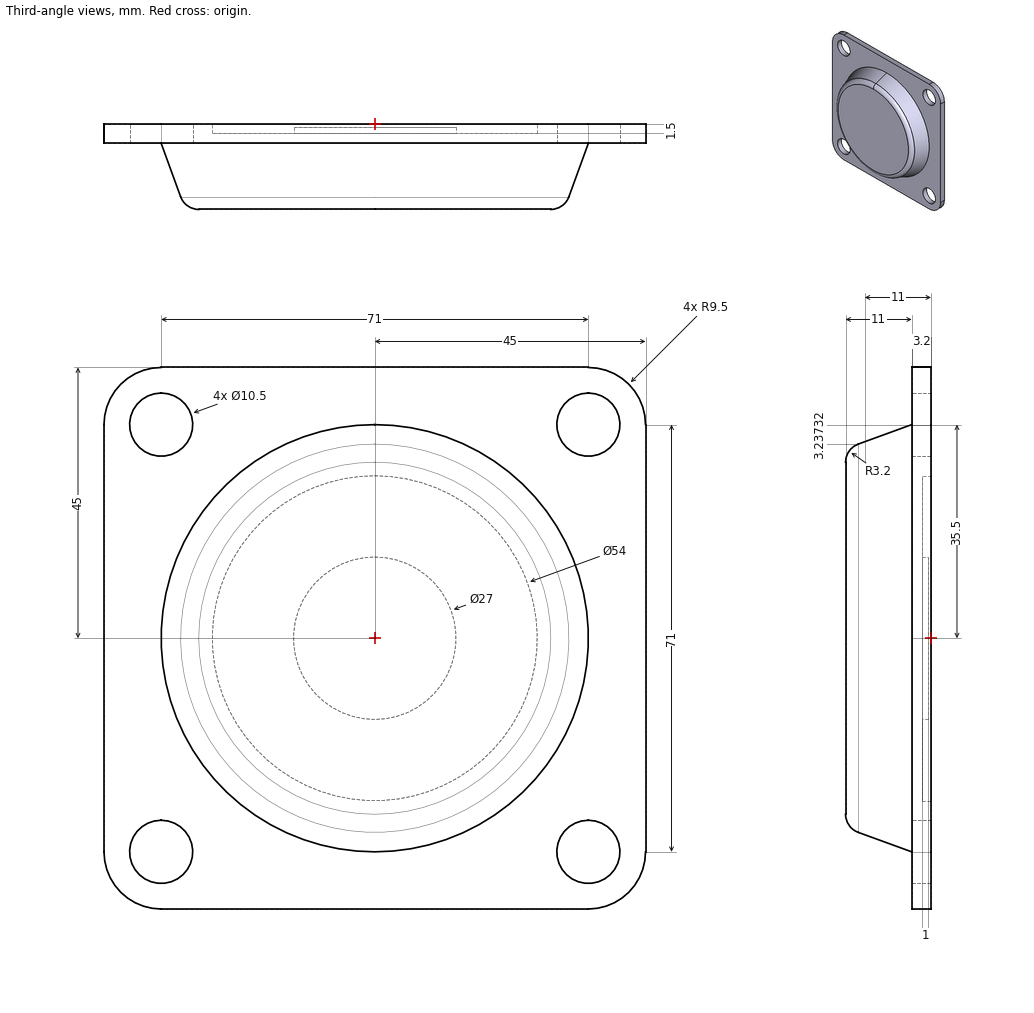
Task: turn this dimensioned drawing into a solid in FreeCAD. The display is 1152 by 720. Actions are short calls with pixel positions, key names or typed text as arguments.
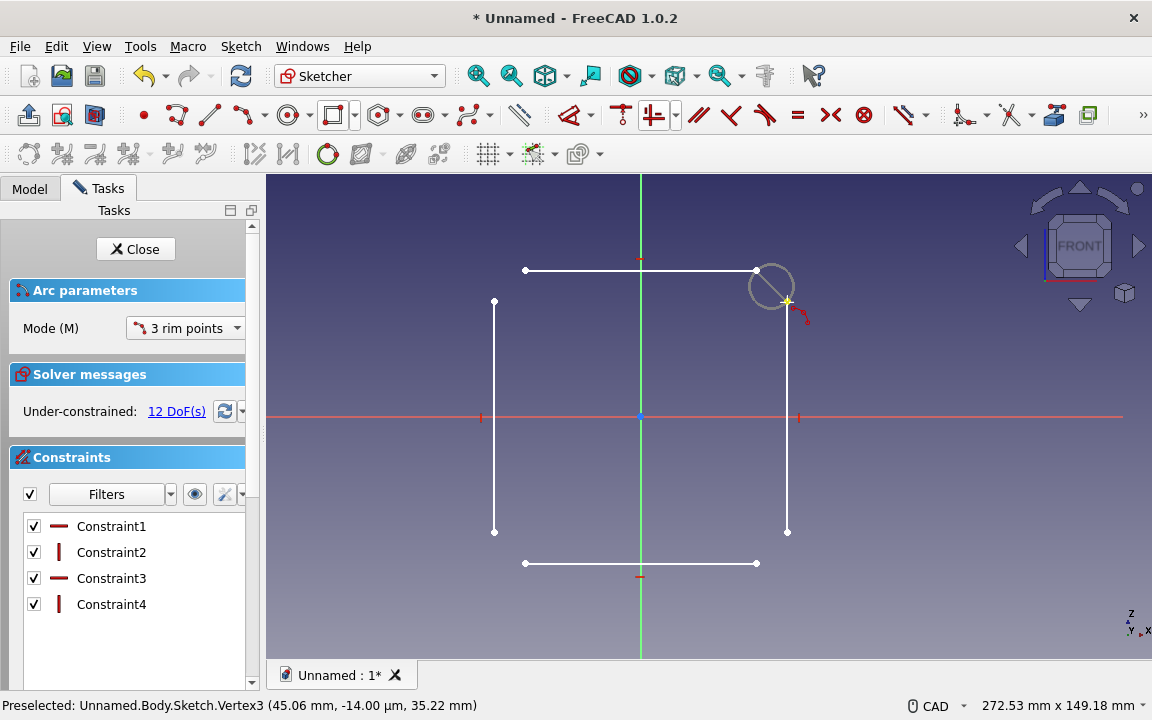
scroll(778, 279, up, 3)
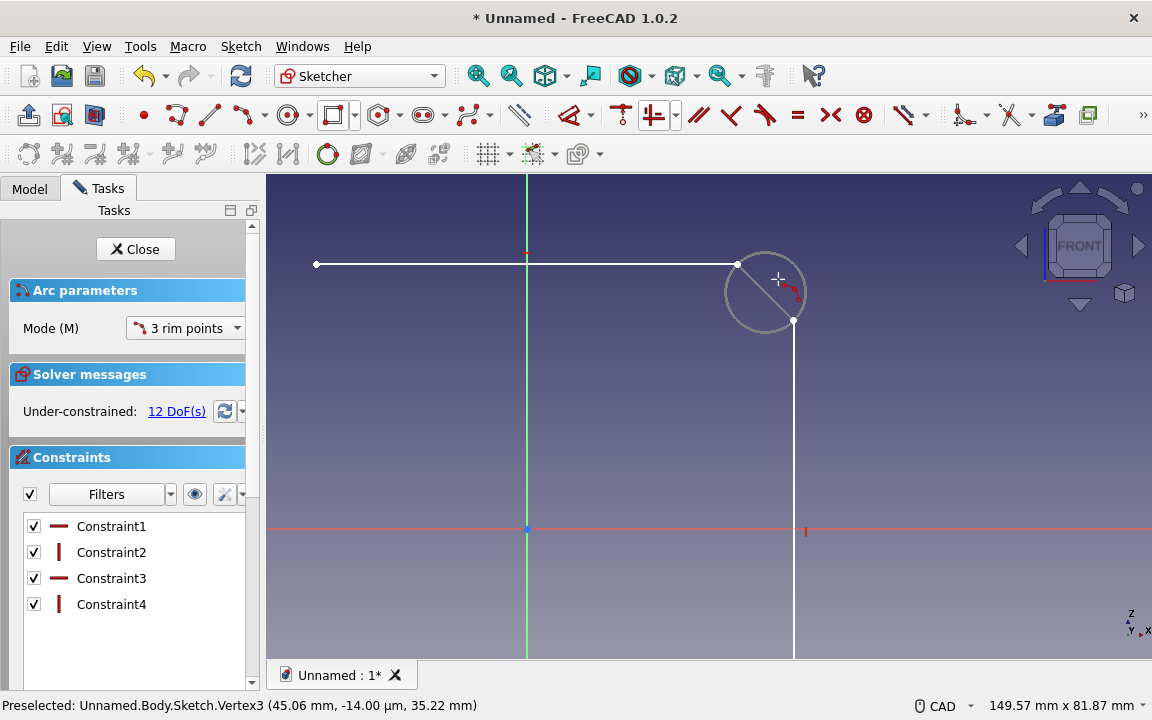
click(777, 279)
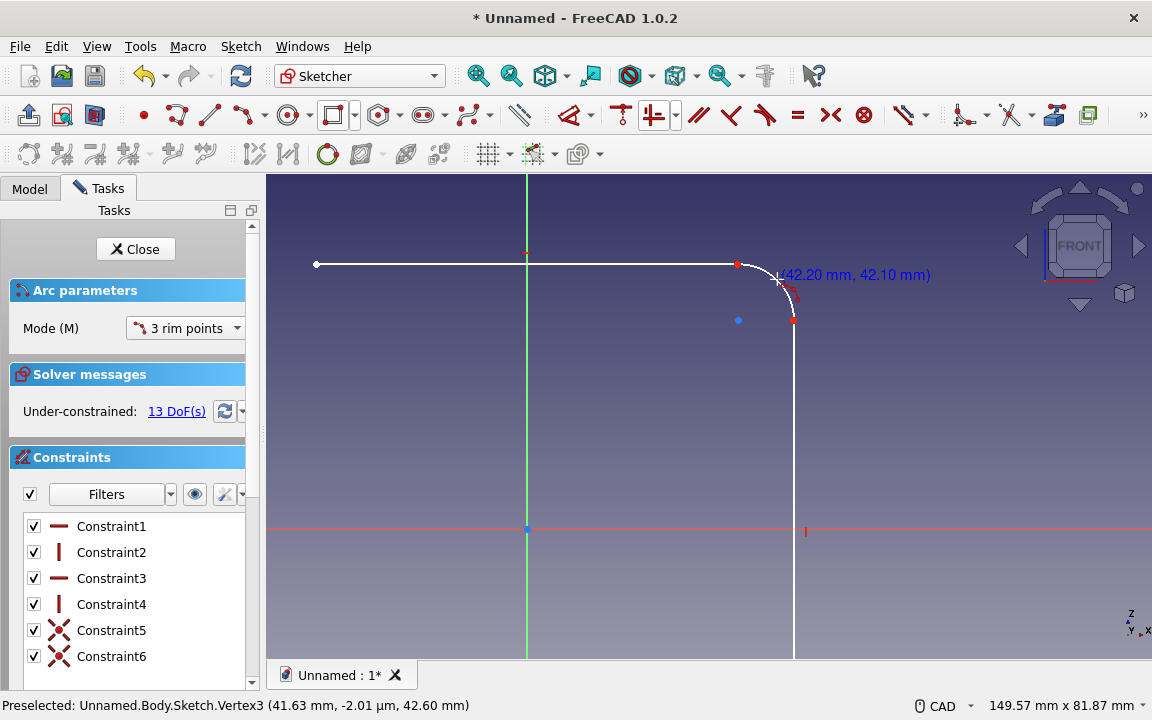
scroll(779, 279, down, 3)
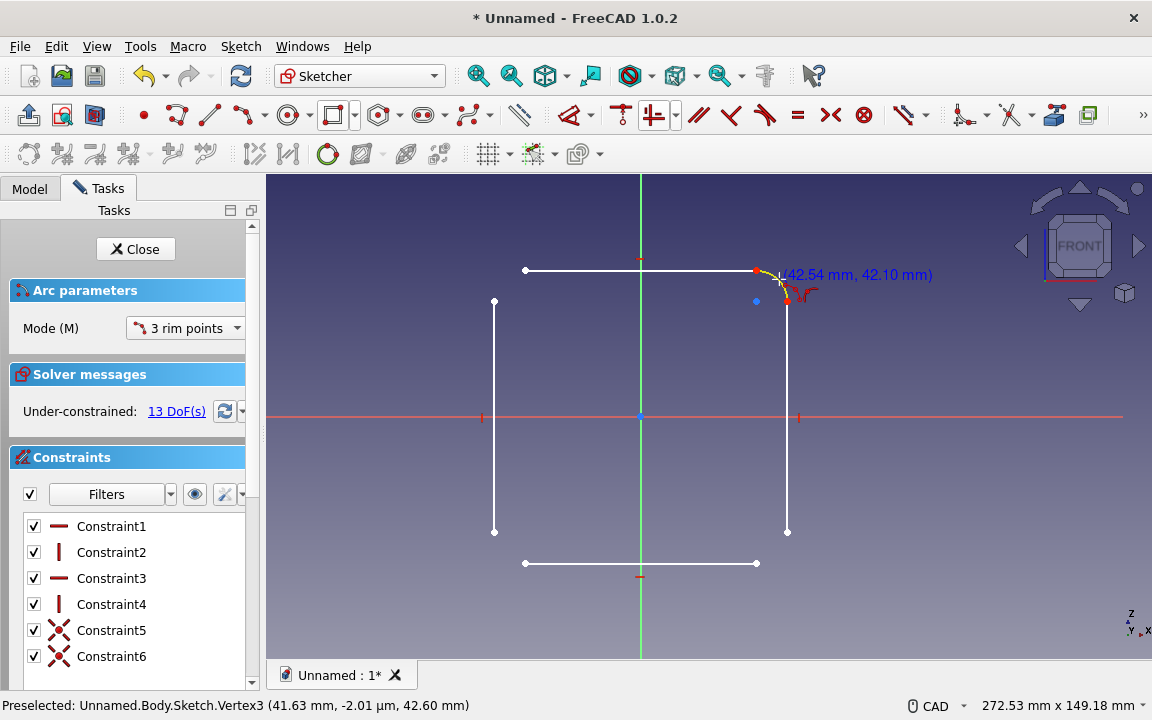
click(787, 533)
click(756, 564)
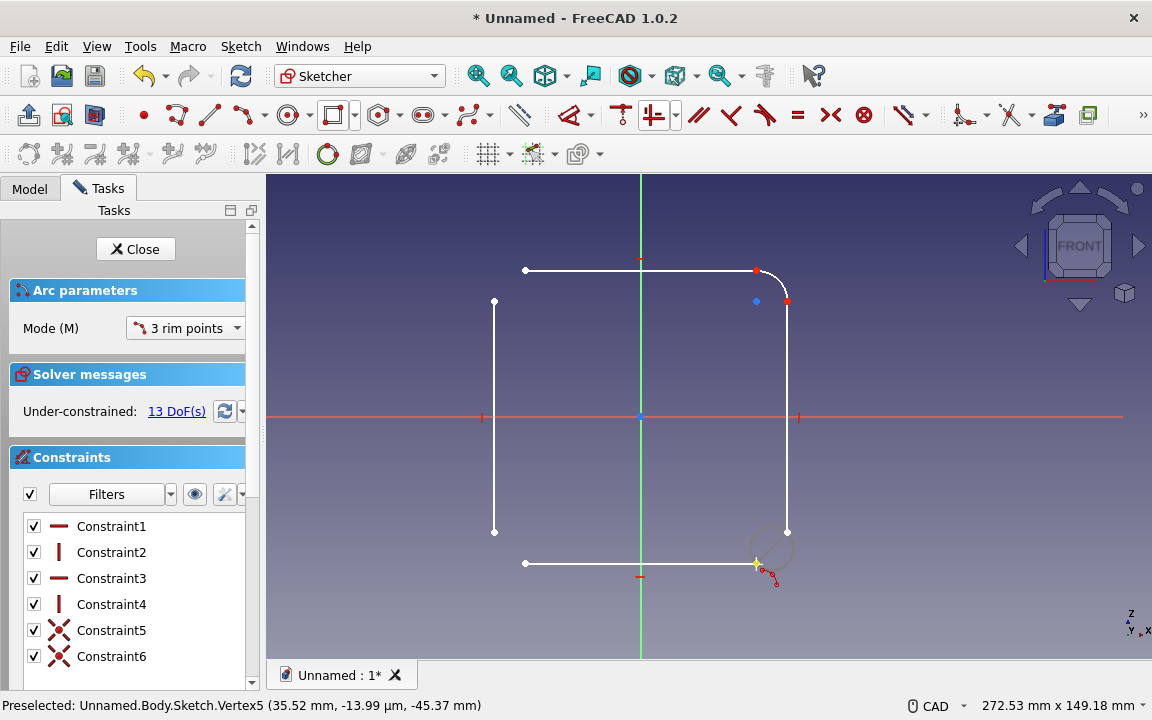
scroll(778, 554, up, 3)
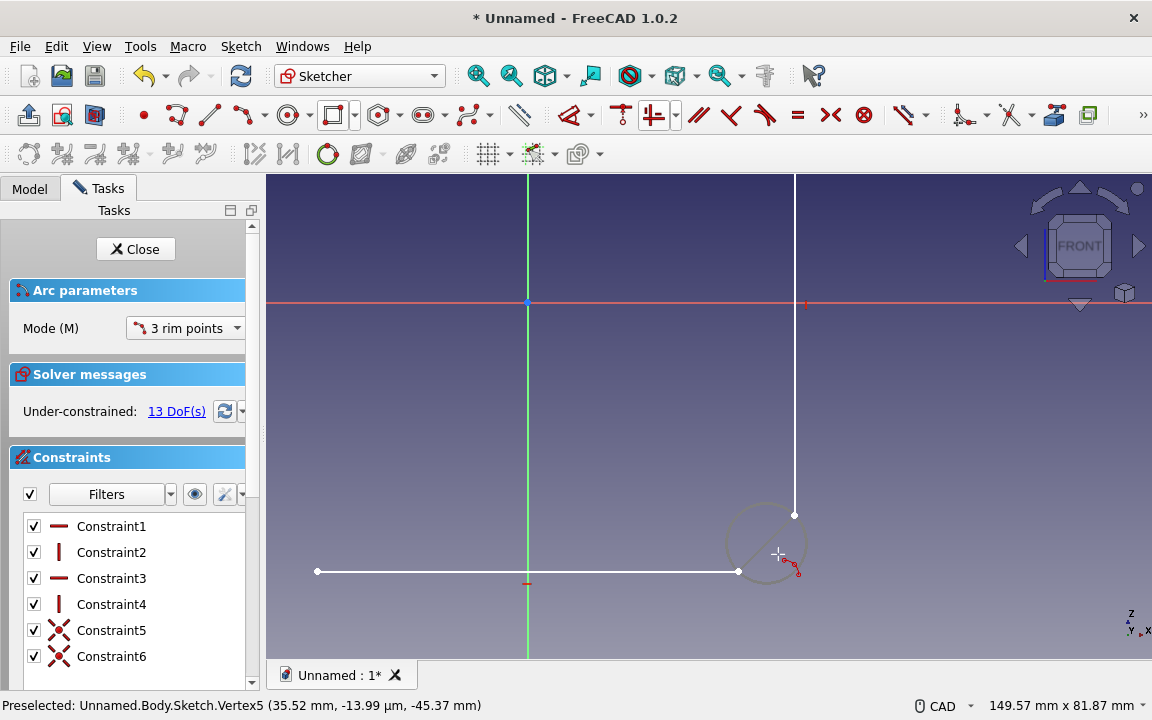
click(778, 553)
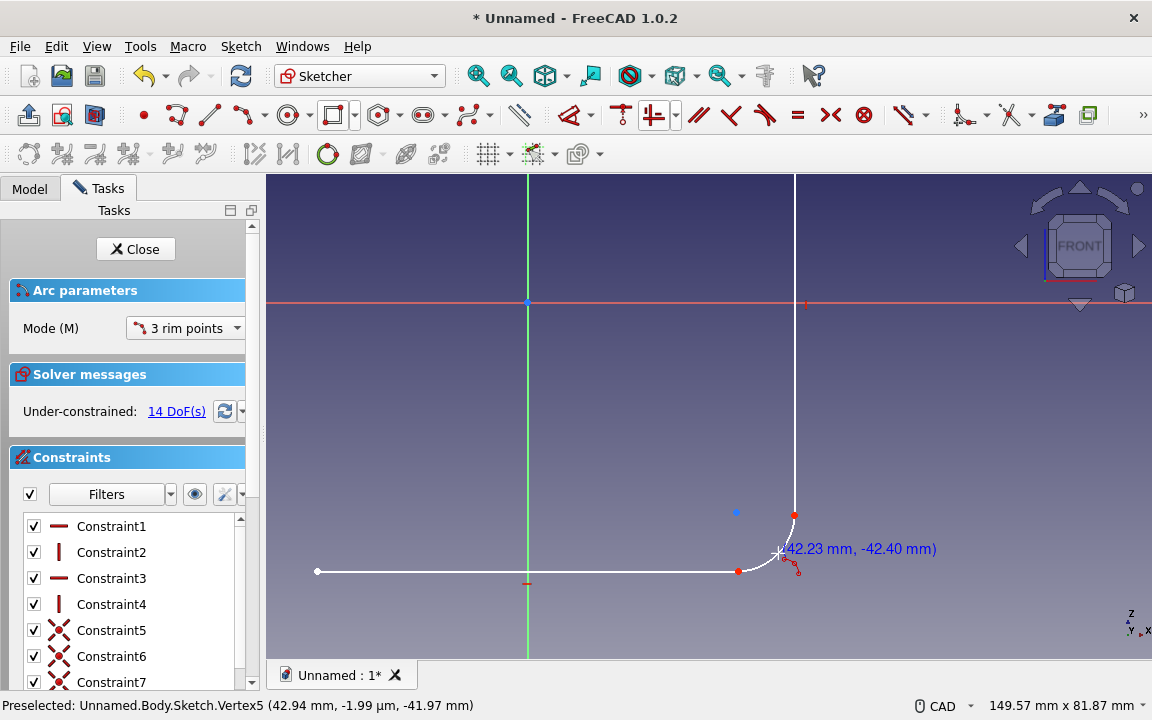
click(317, 572)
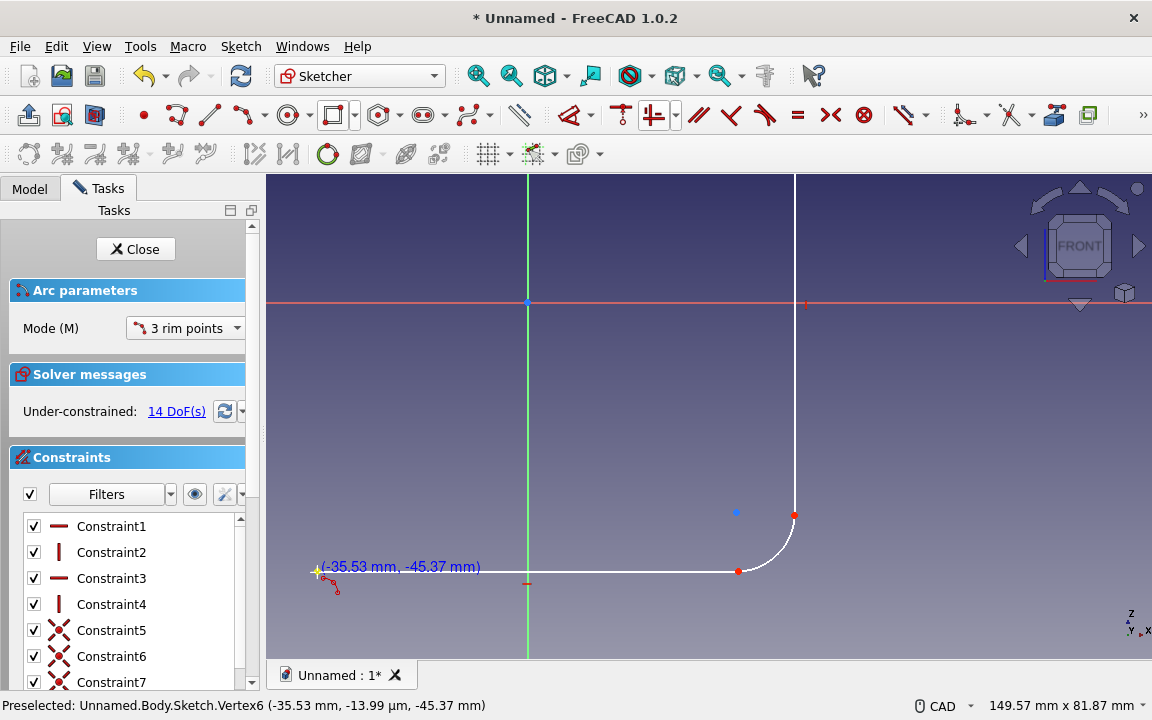
scroll(778, 555, down, 3)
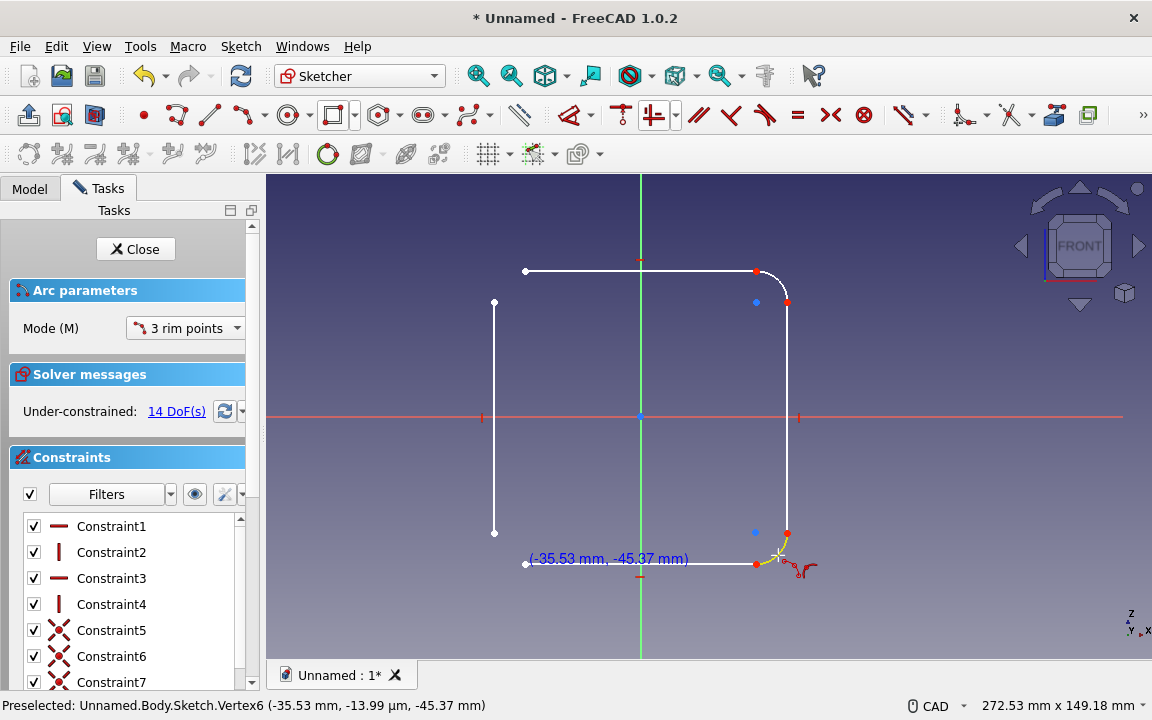
click(494, 533)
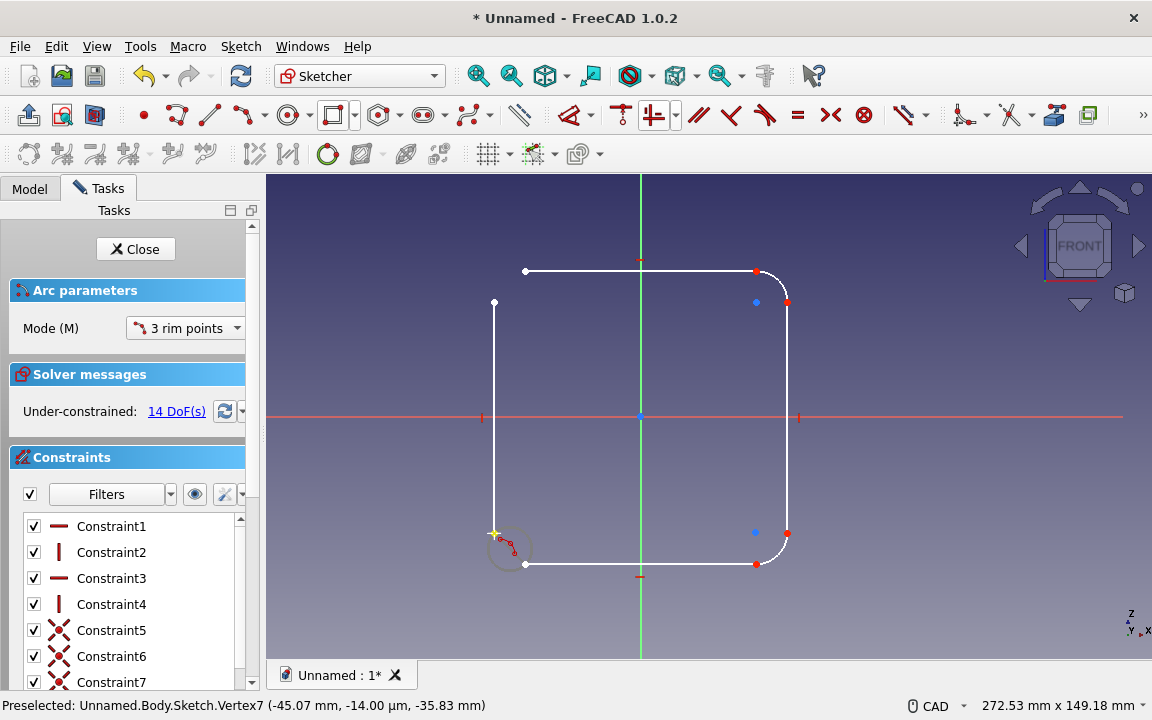
scroll(504, 554, up, 3)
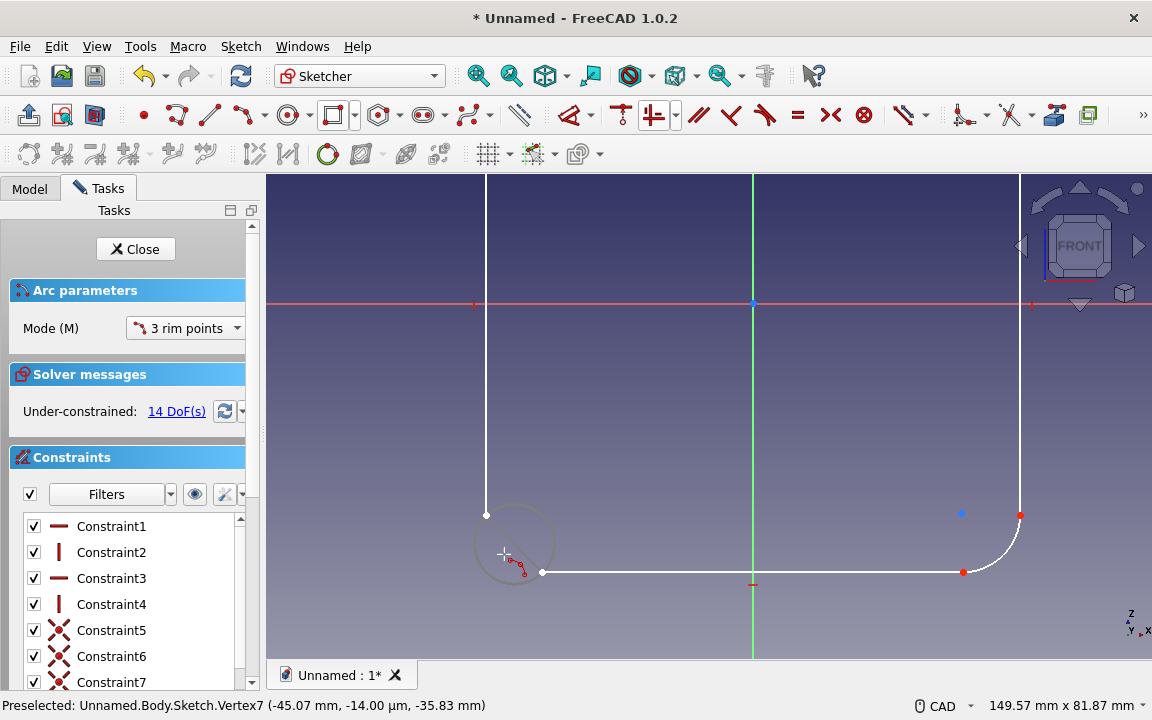
click(503, 554)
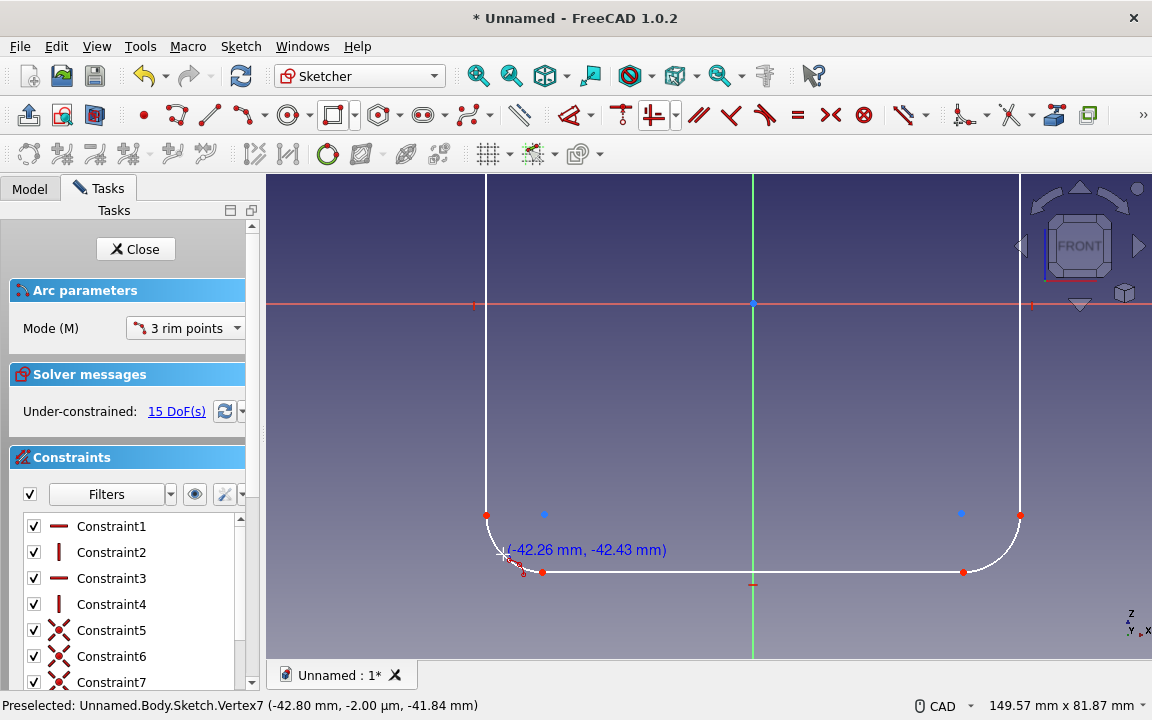
scroll(503, 554, down, 3)